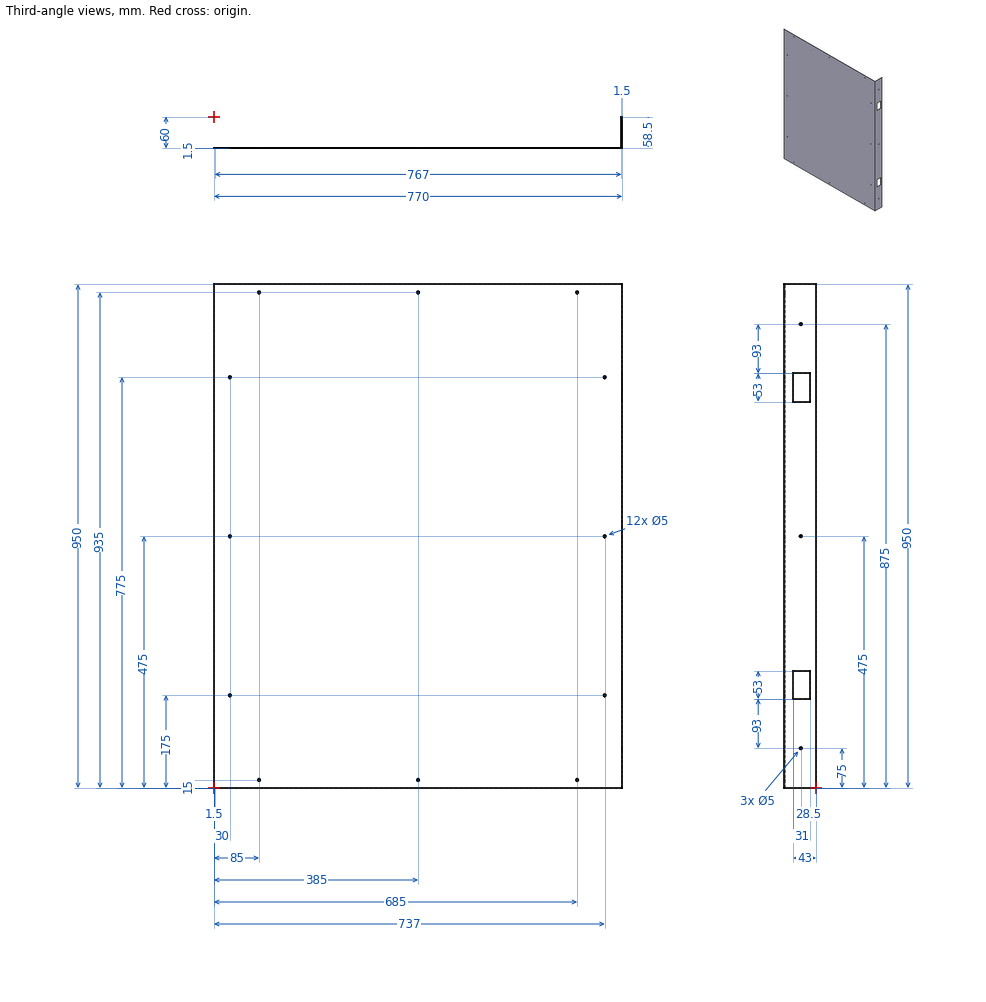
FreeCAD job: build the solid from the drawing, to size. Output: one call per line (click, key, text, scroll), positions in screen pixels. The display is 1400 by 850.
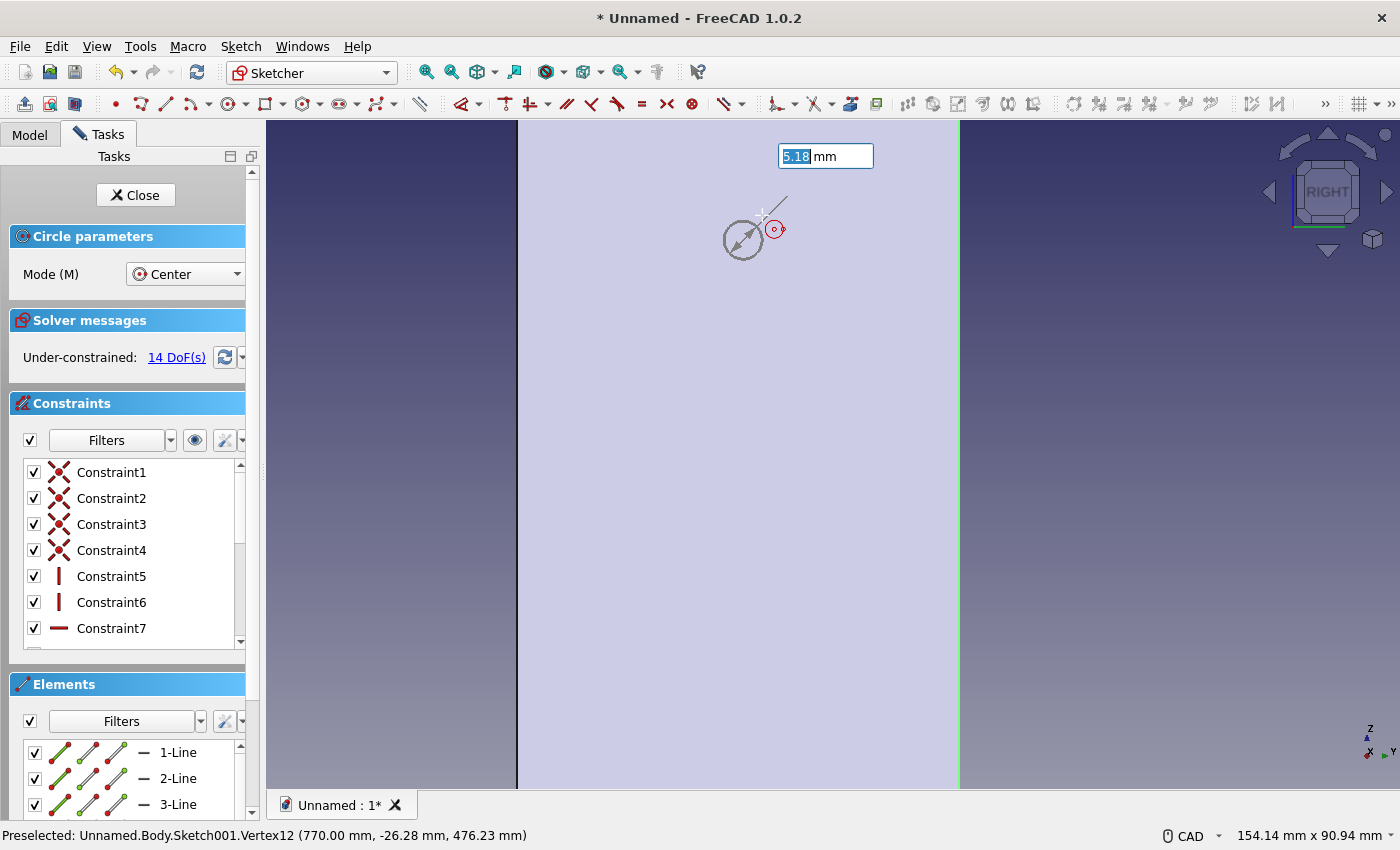
click(762, 213)
key(Escape)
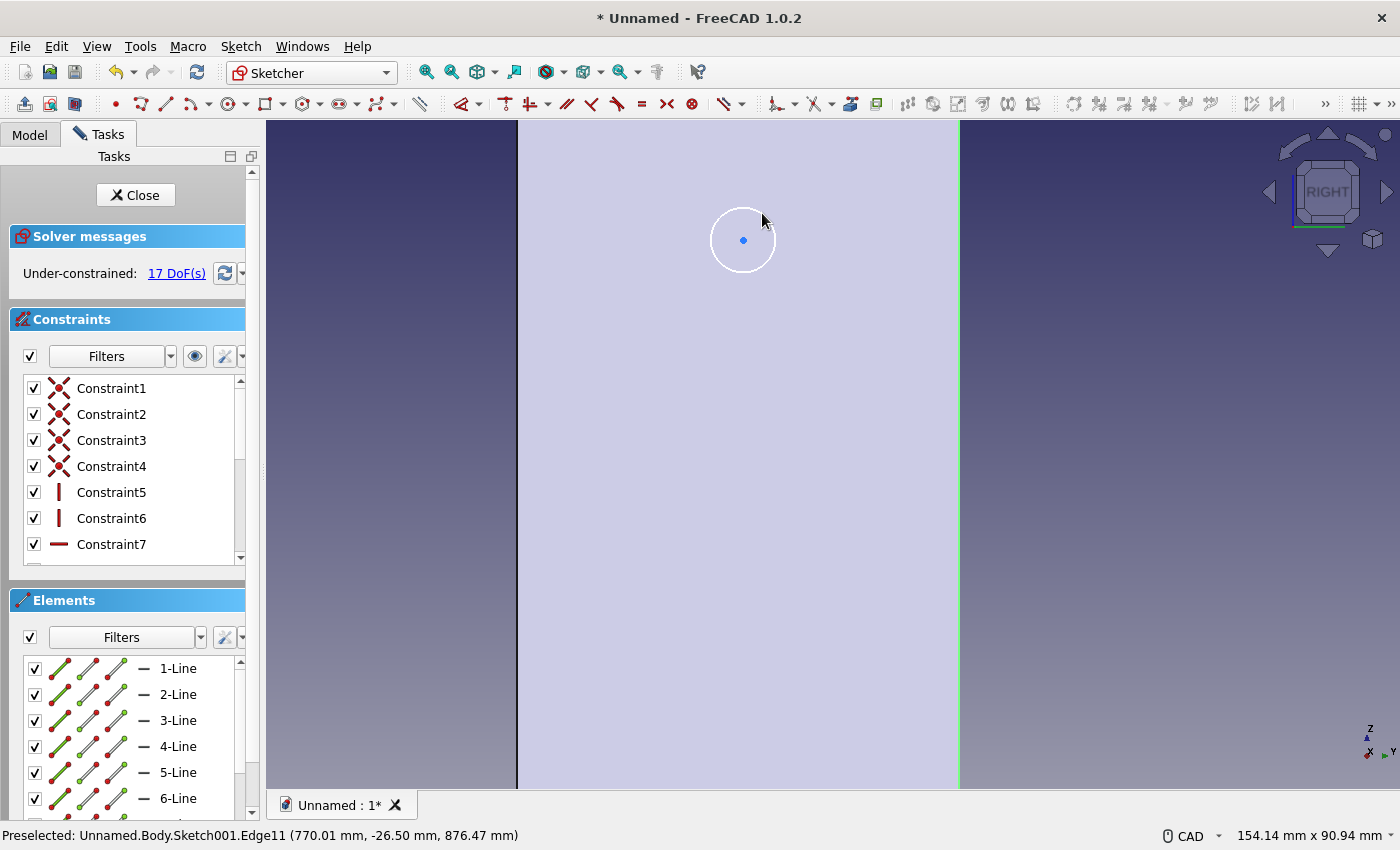
scroll(762, 261, down, 14)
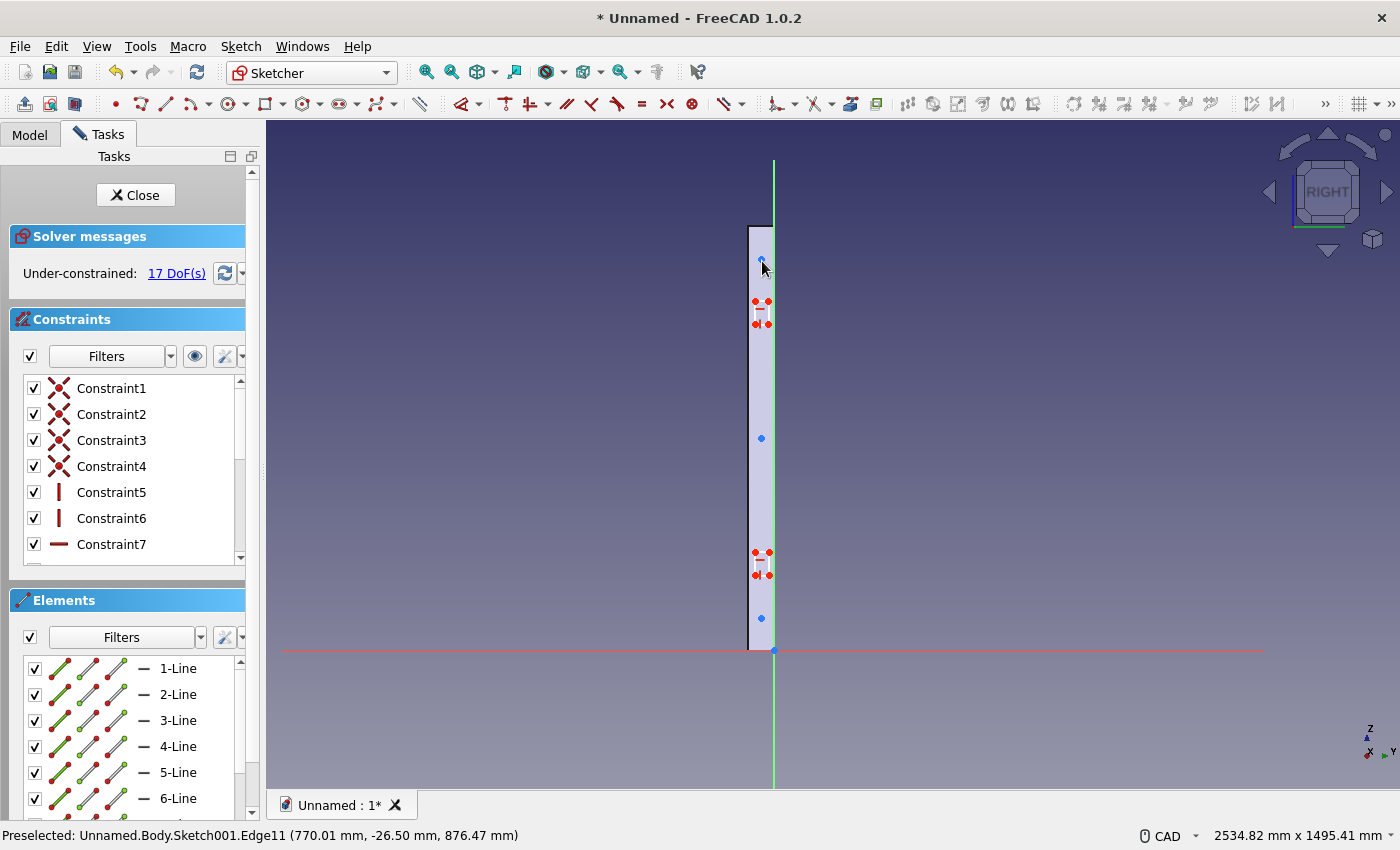
scroll(763, 617, up, 10)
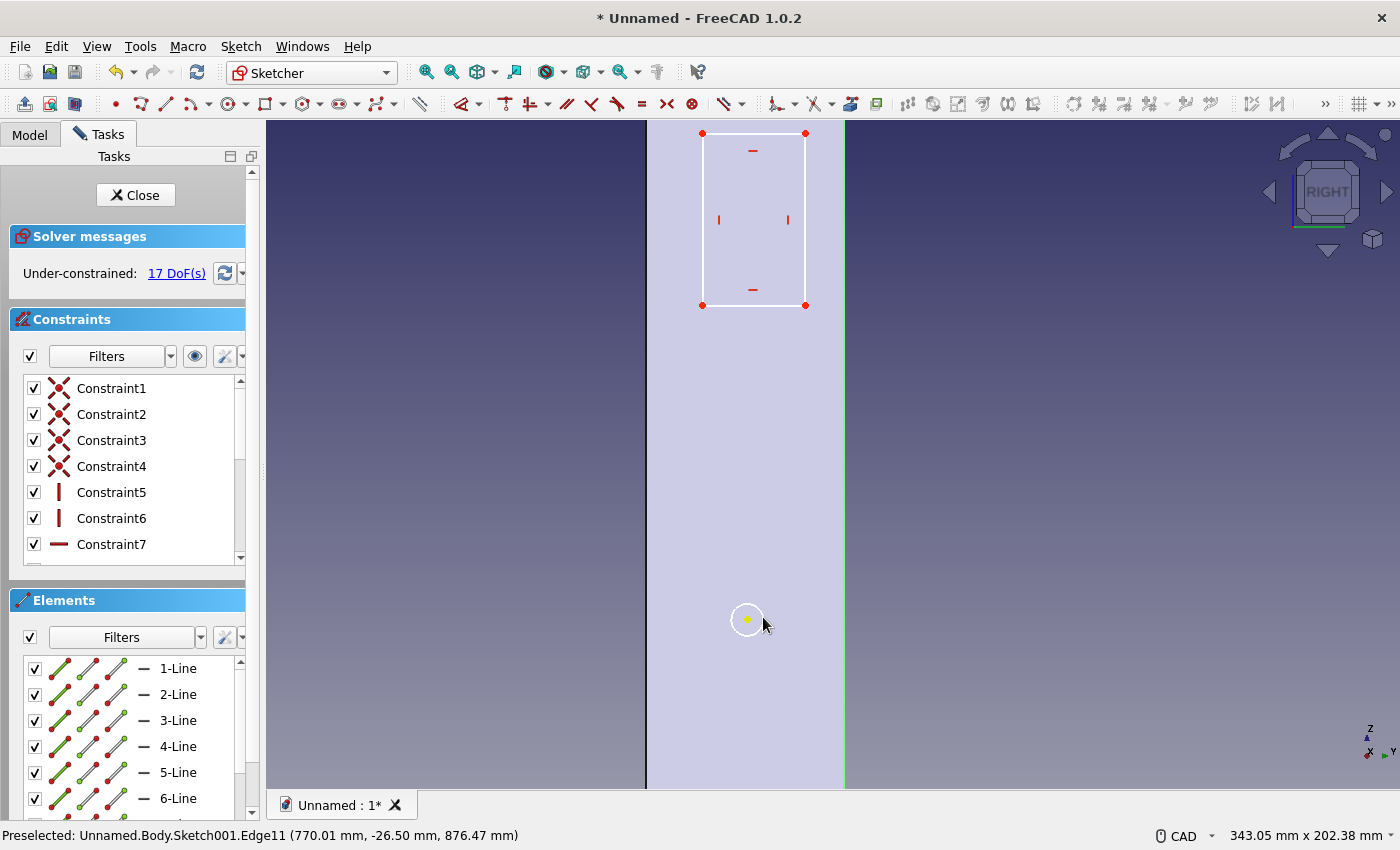
click(759, 609)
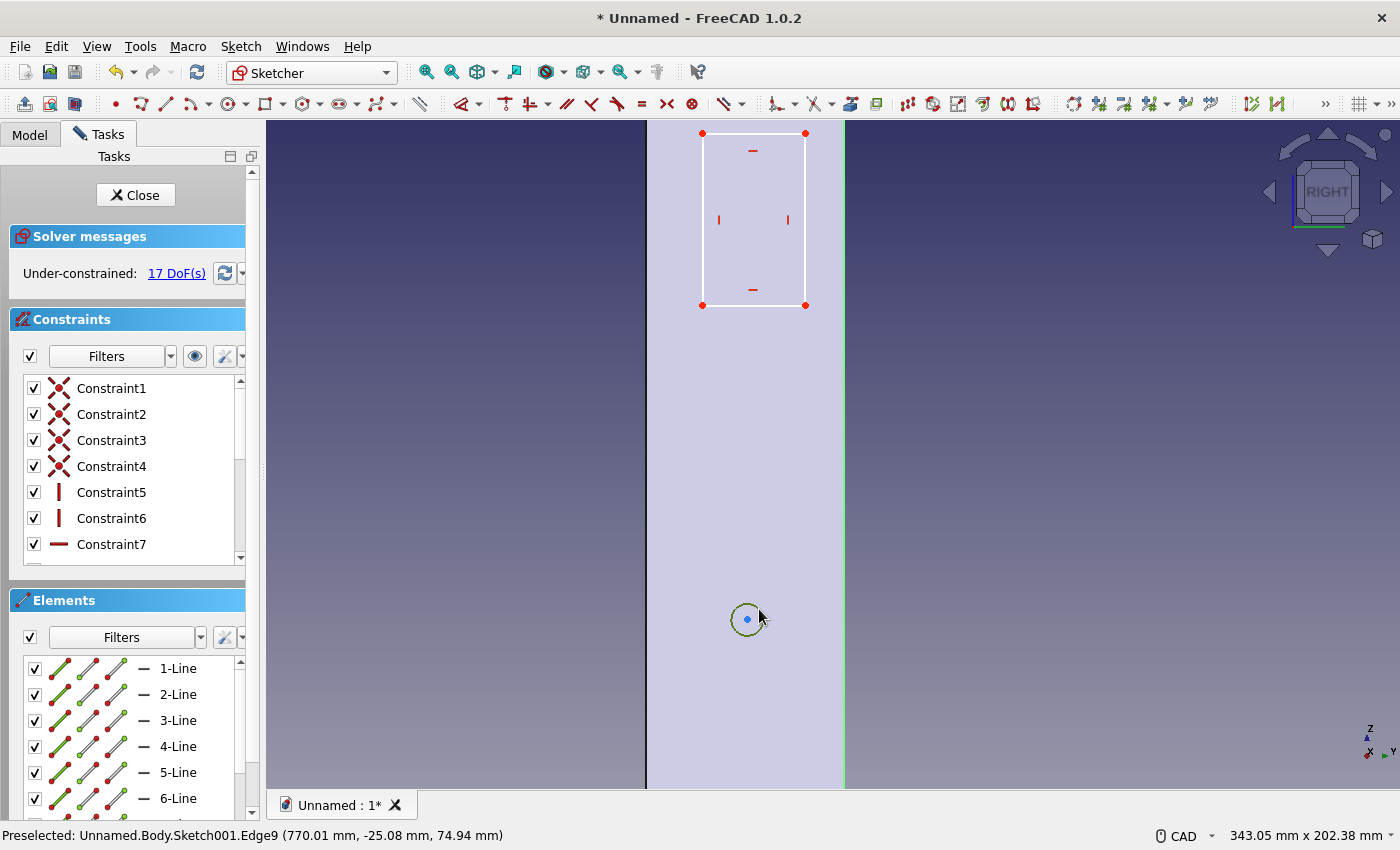
scroll(763, 618, down, 10)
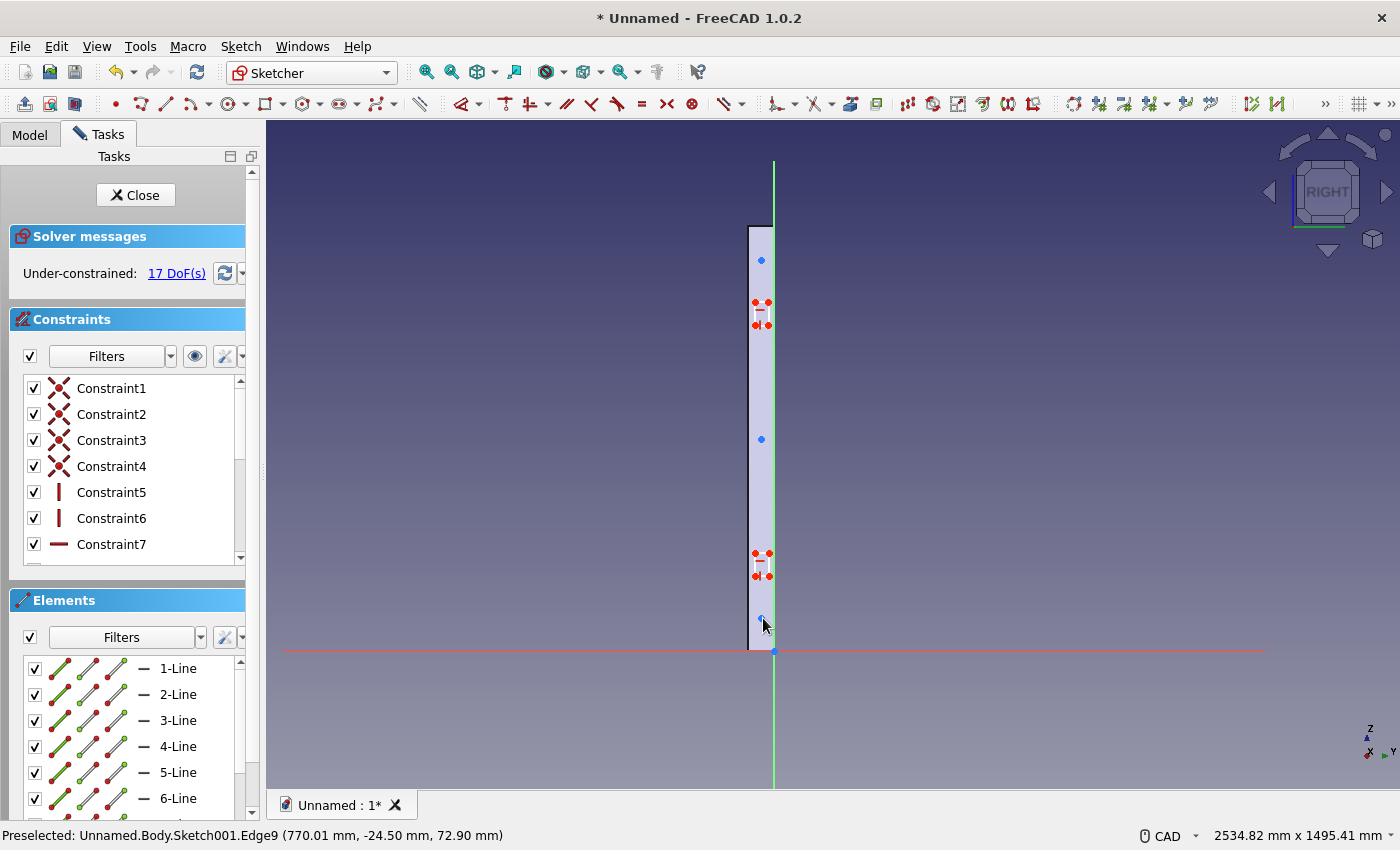
scroll(763, 438, up, 11)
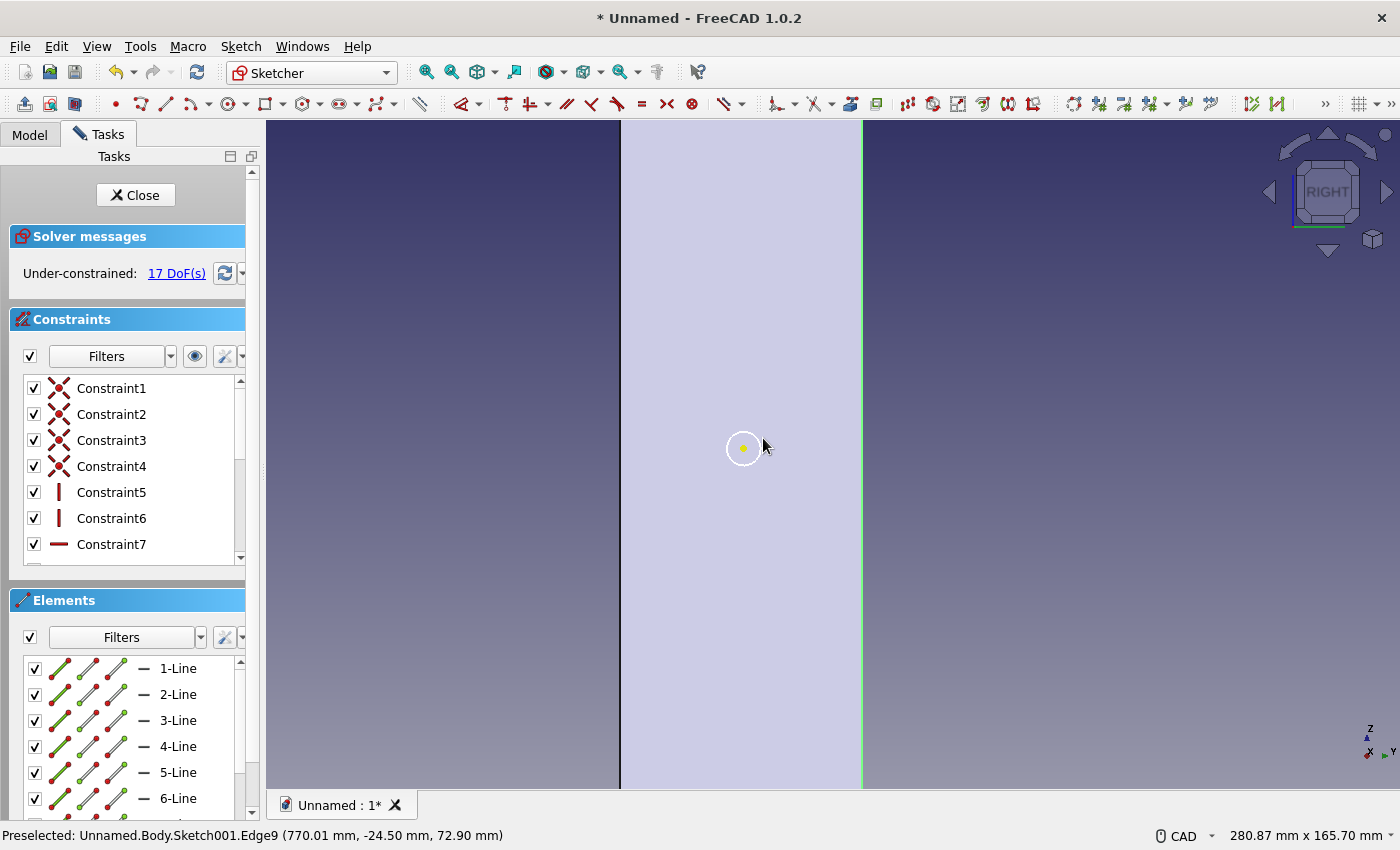
click(756, 437)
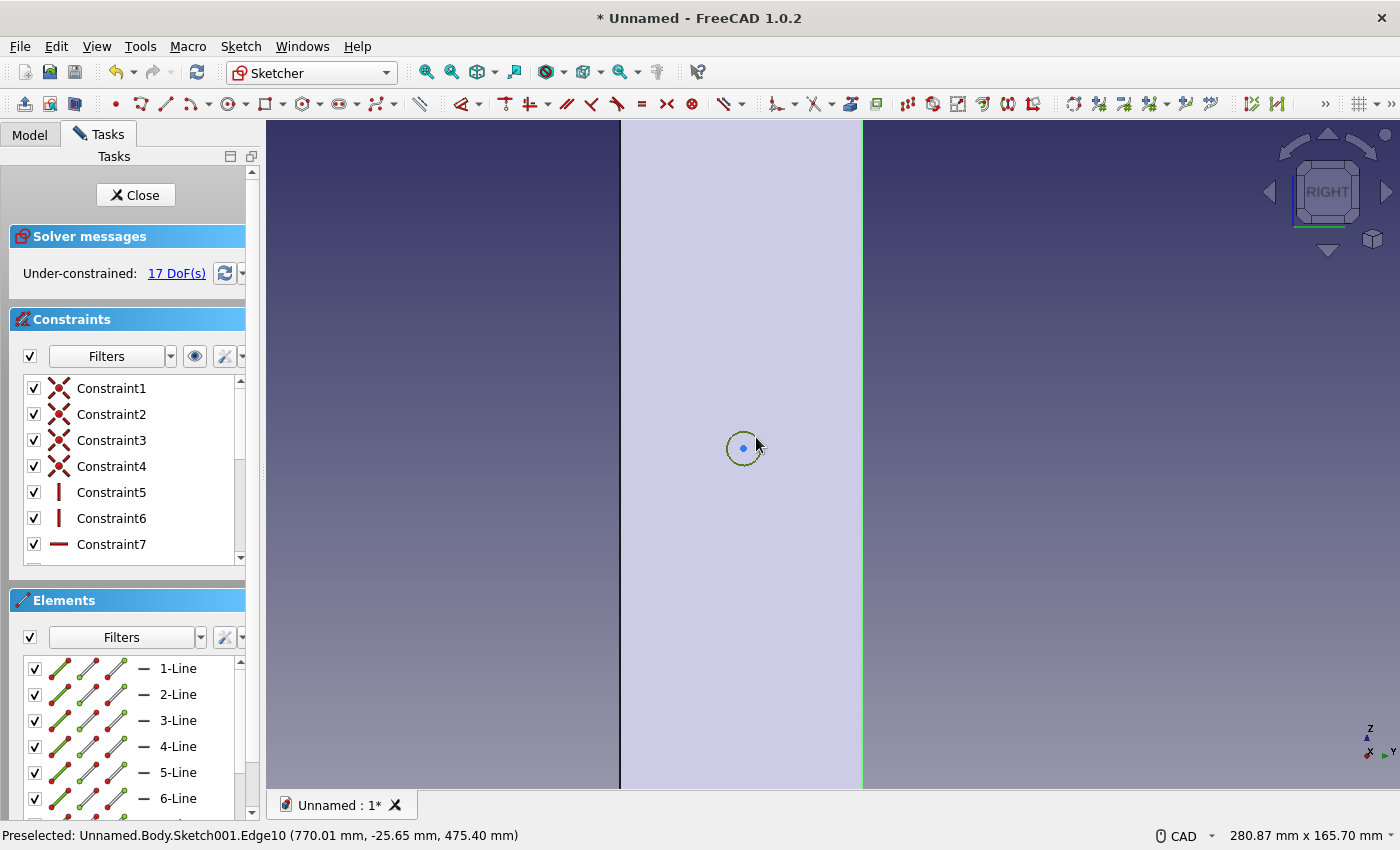
scroll(763, 438, down, 11)